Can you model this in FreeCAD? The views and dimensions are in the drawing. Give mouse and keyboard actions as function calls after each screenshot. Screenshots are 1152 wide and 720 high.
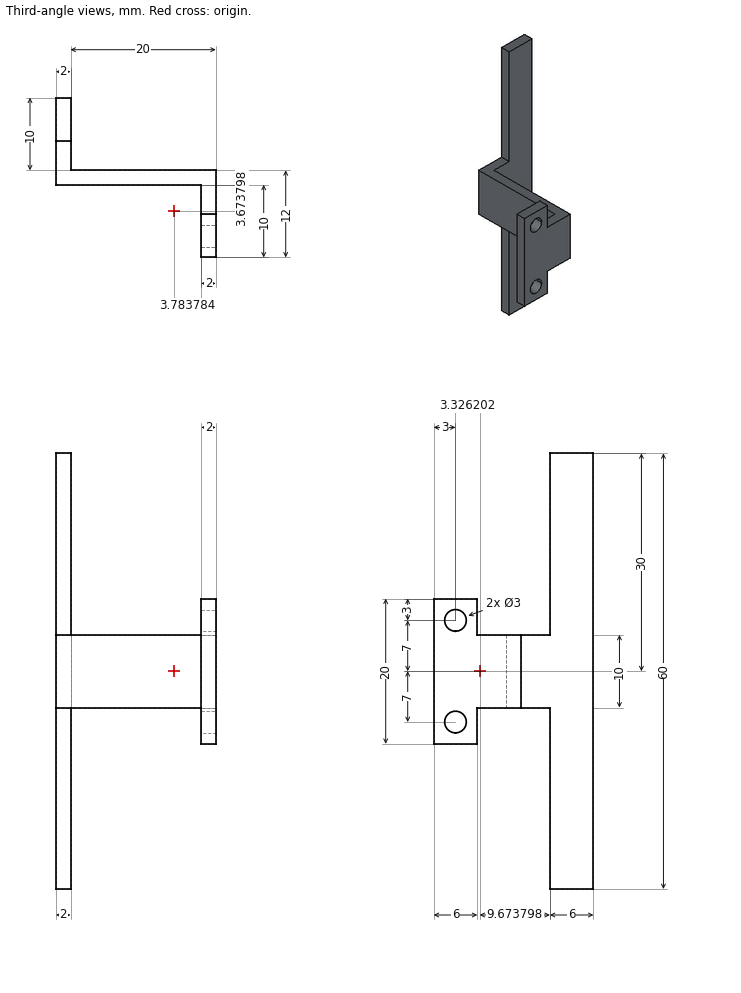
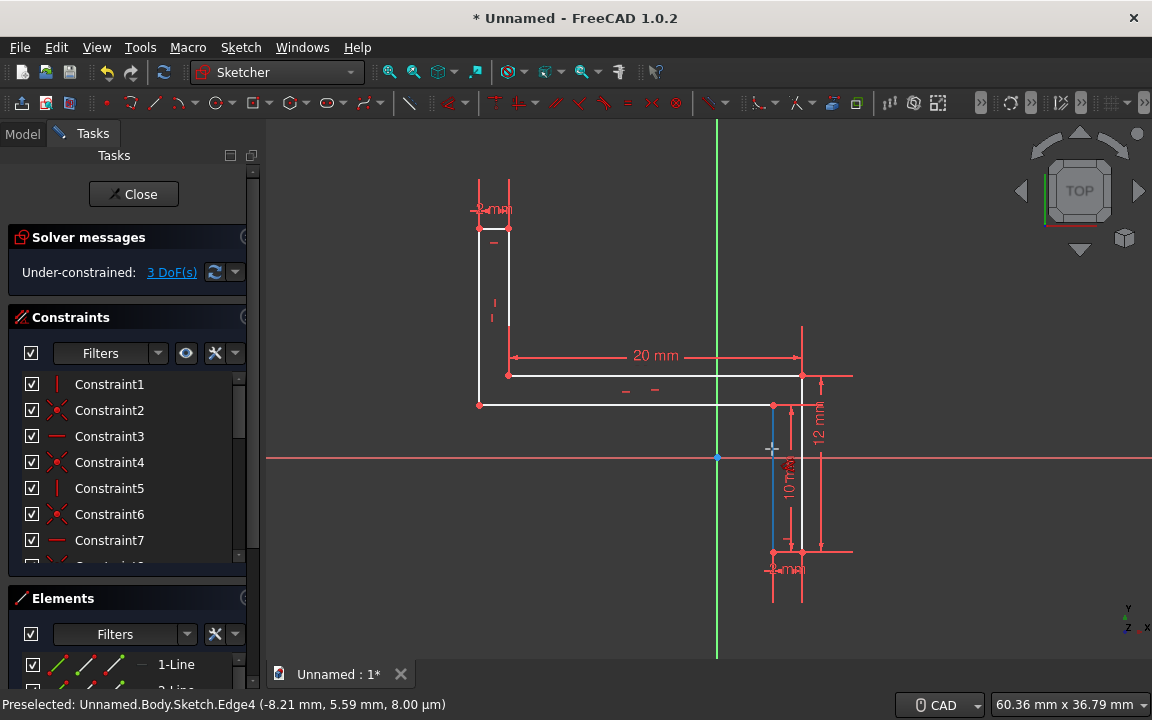
click(509, 332)
click(543, 302)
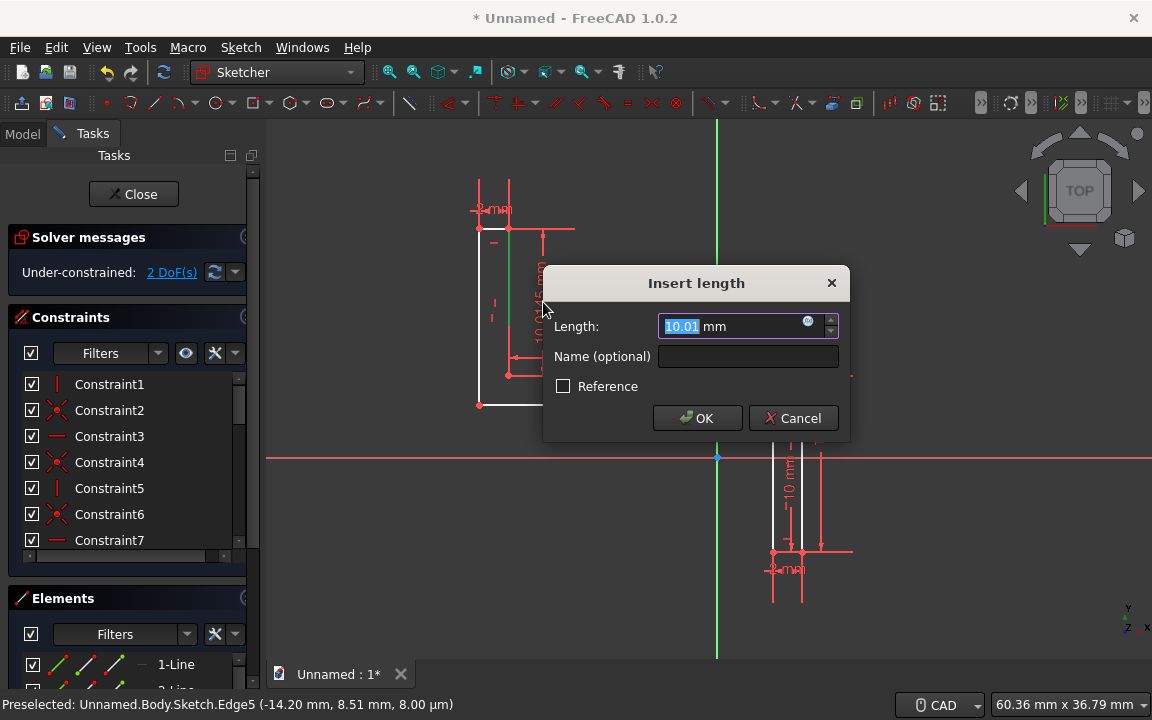
text(10)
key(Return)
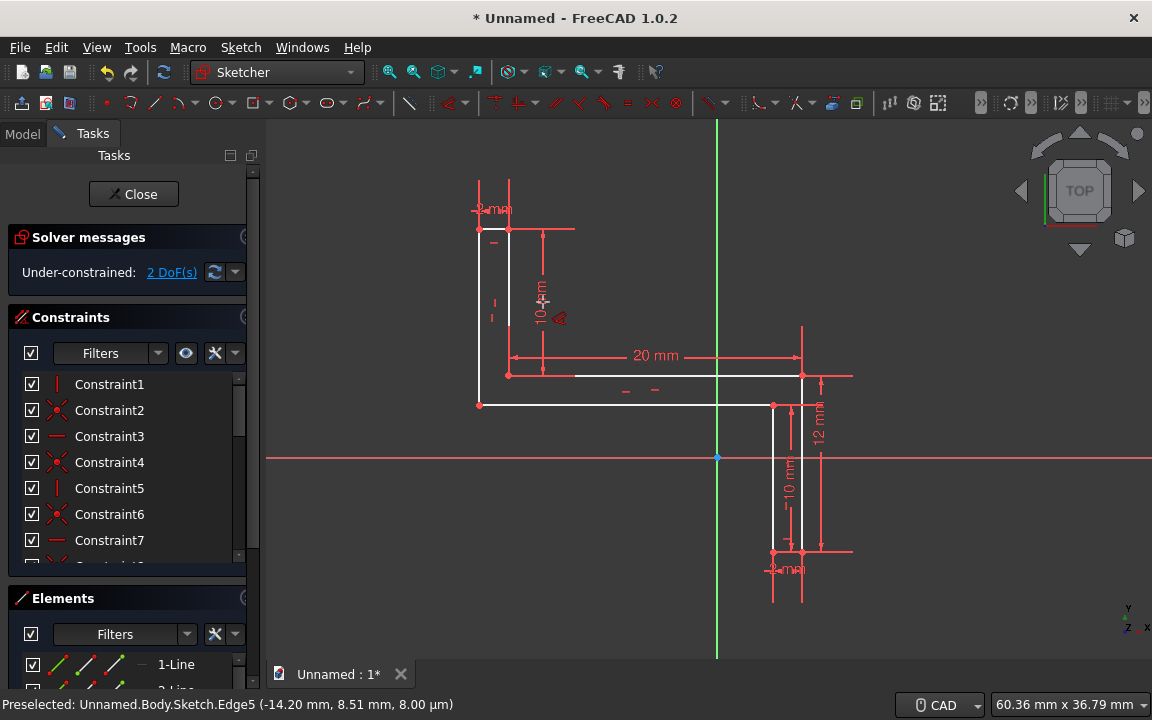
click(773, 405)
click(745, 516)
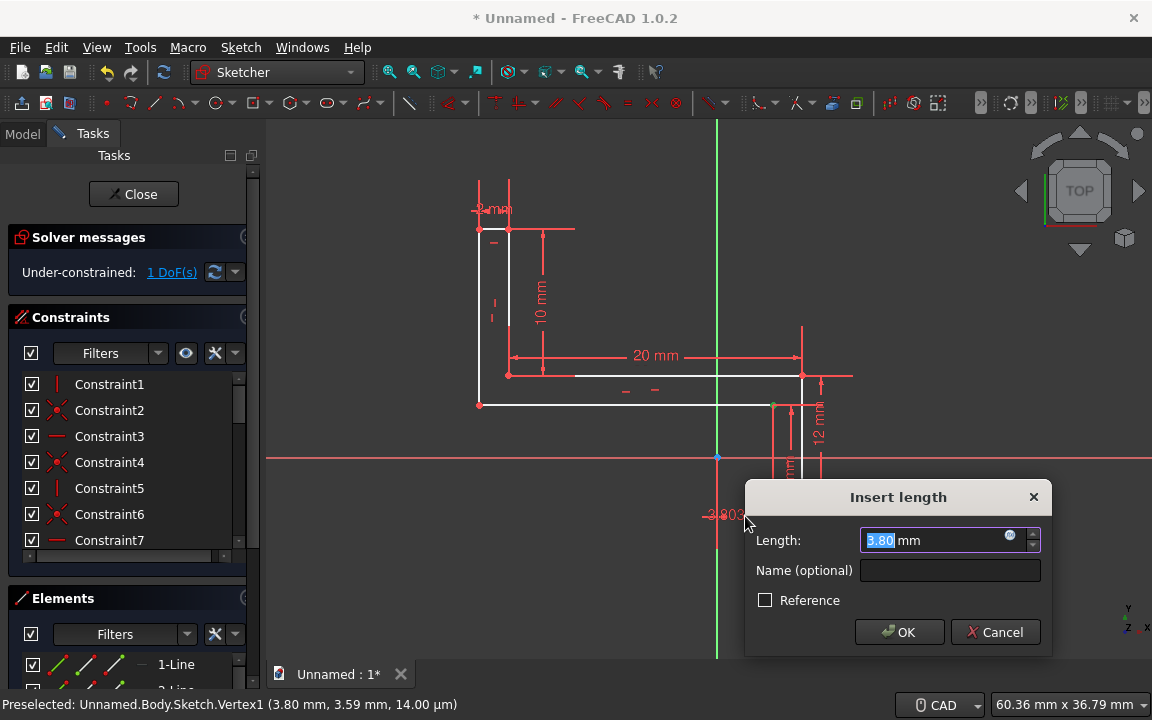
text(3.783784)
key(Return)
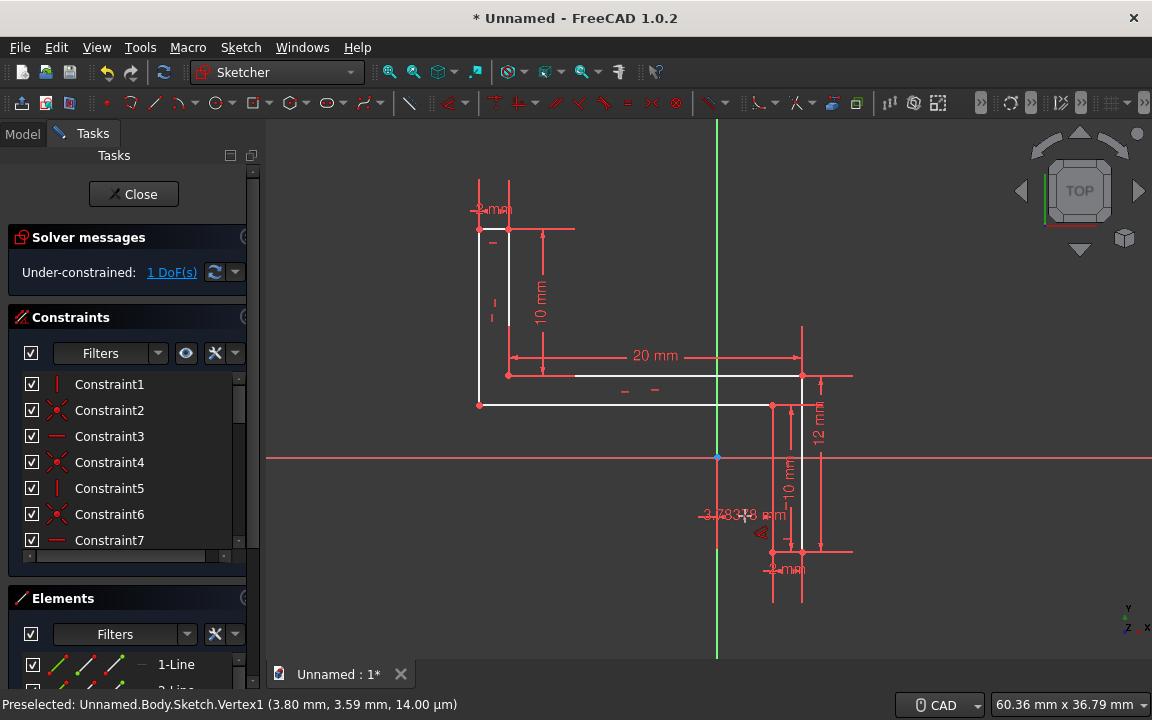
click(773, 405)
click(683, 432)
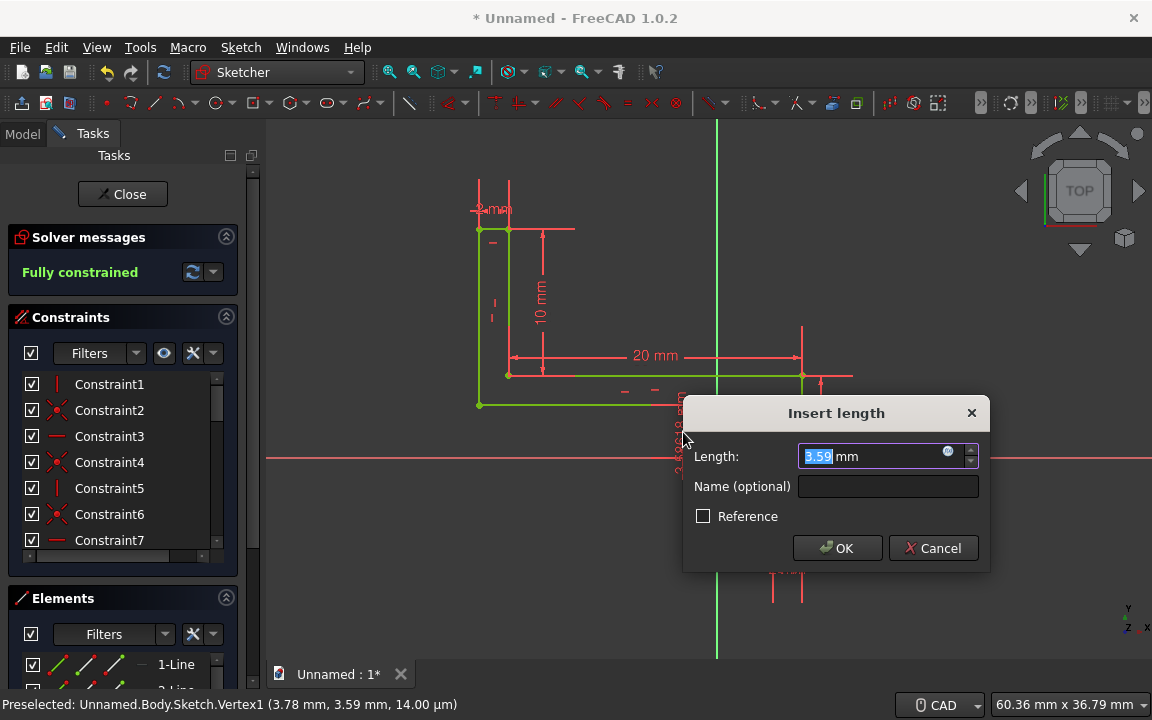
text(3.673798)
key(Return)
key(Escape)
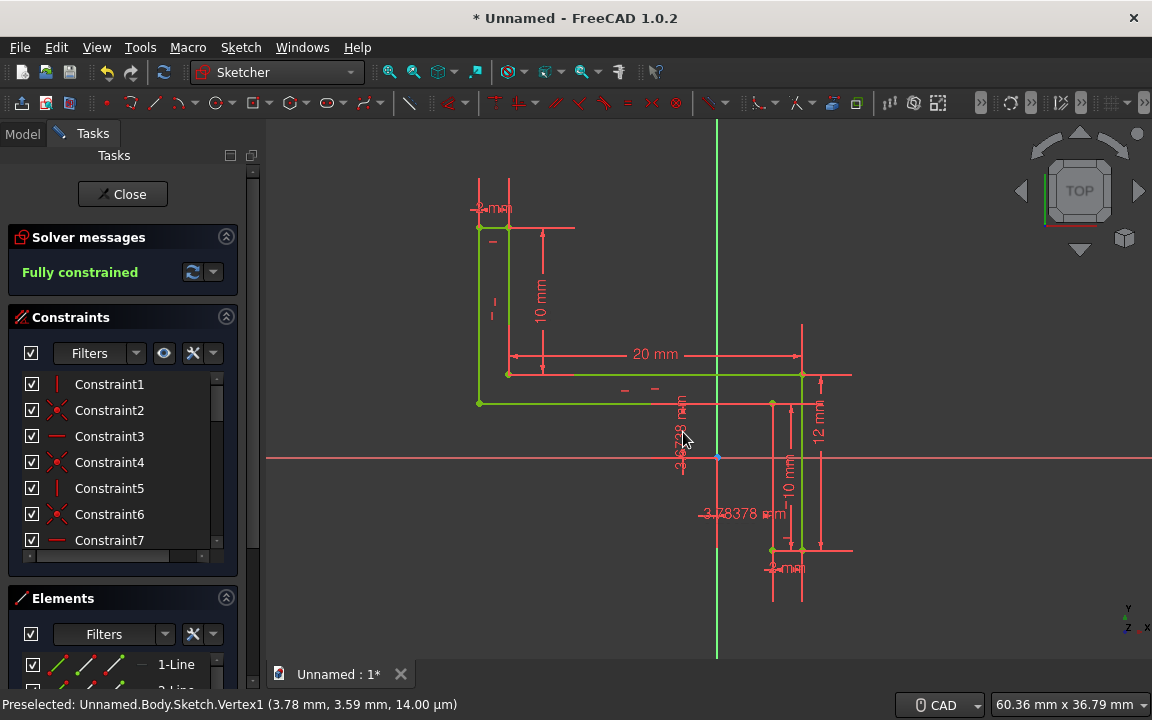
click(123, 194)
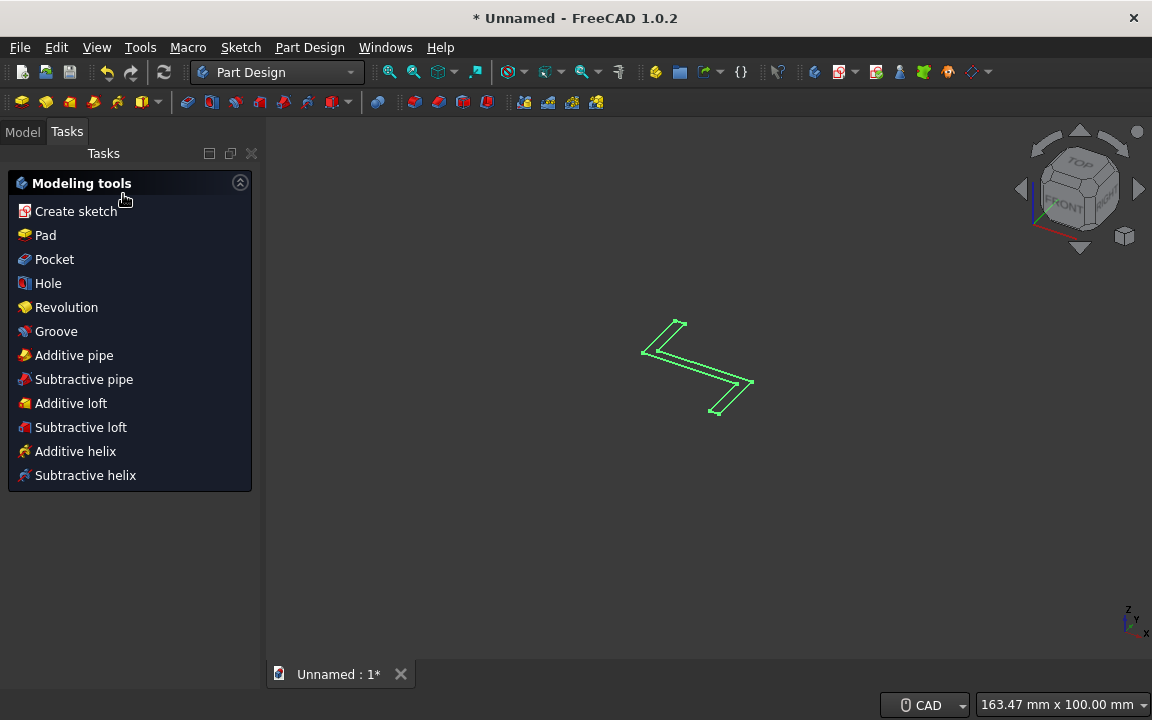
click(22, 102)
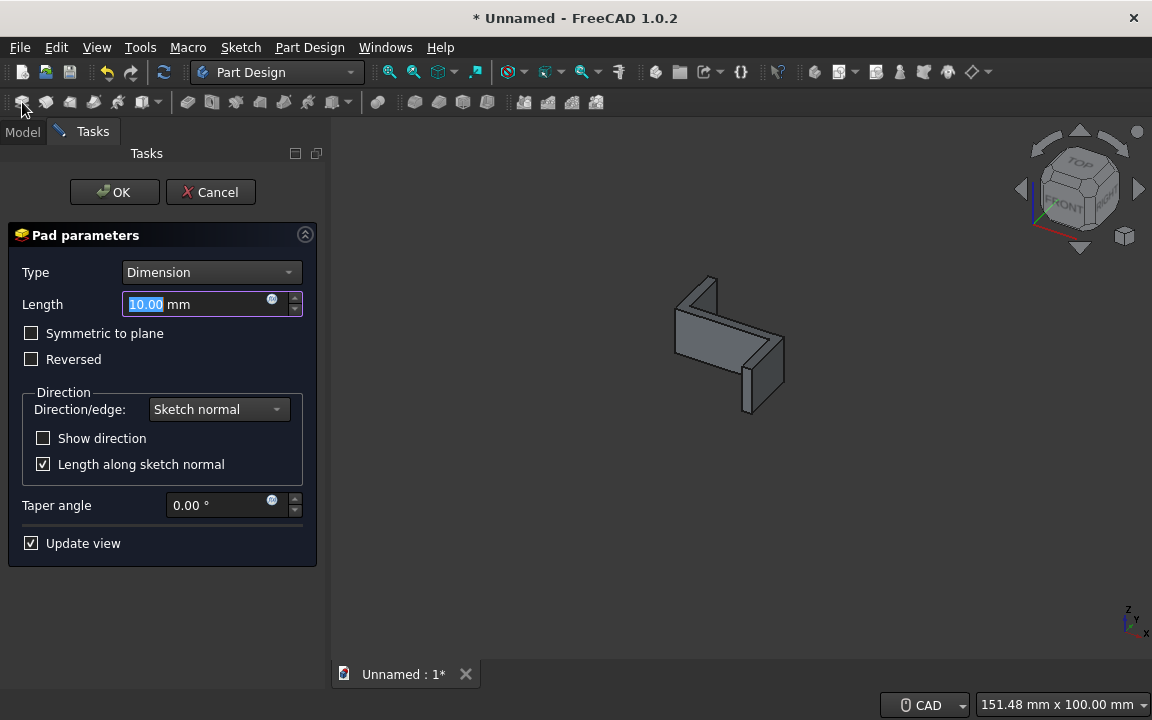
text(10)
key(Tab)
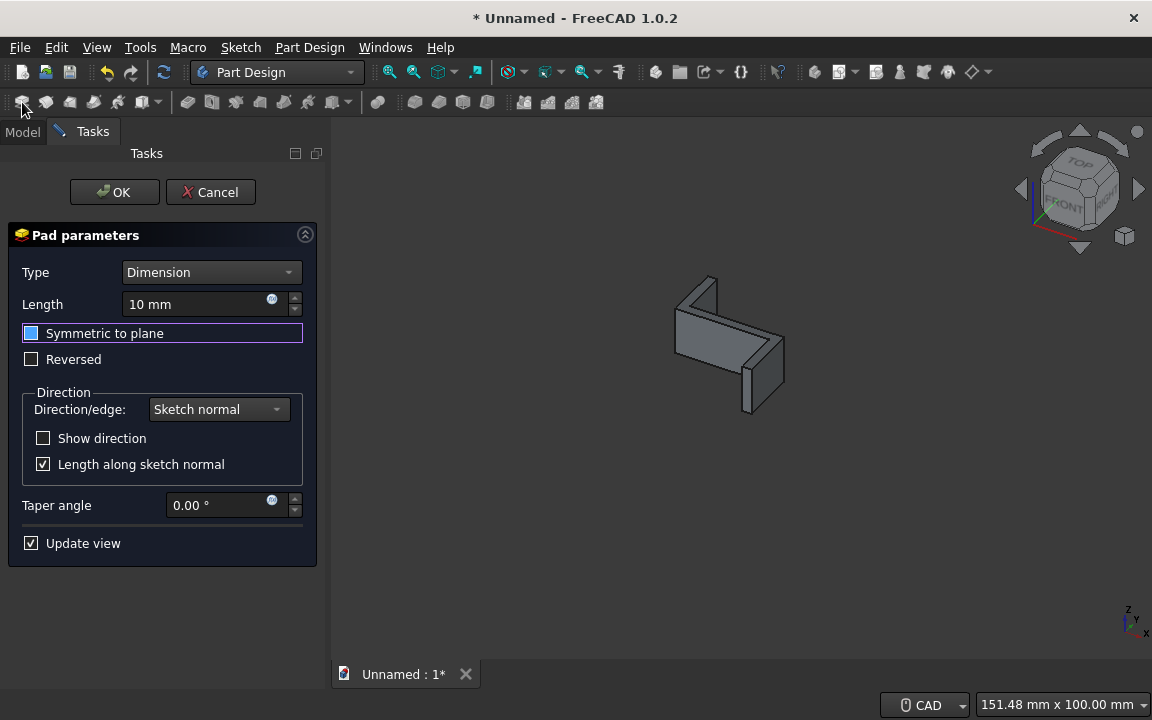
click(30, 333)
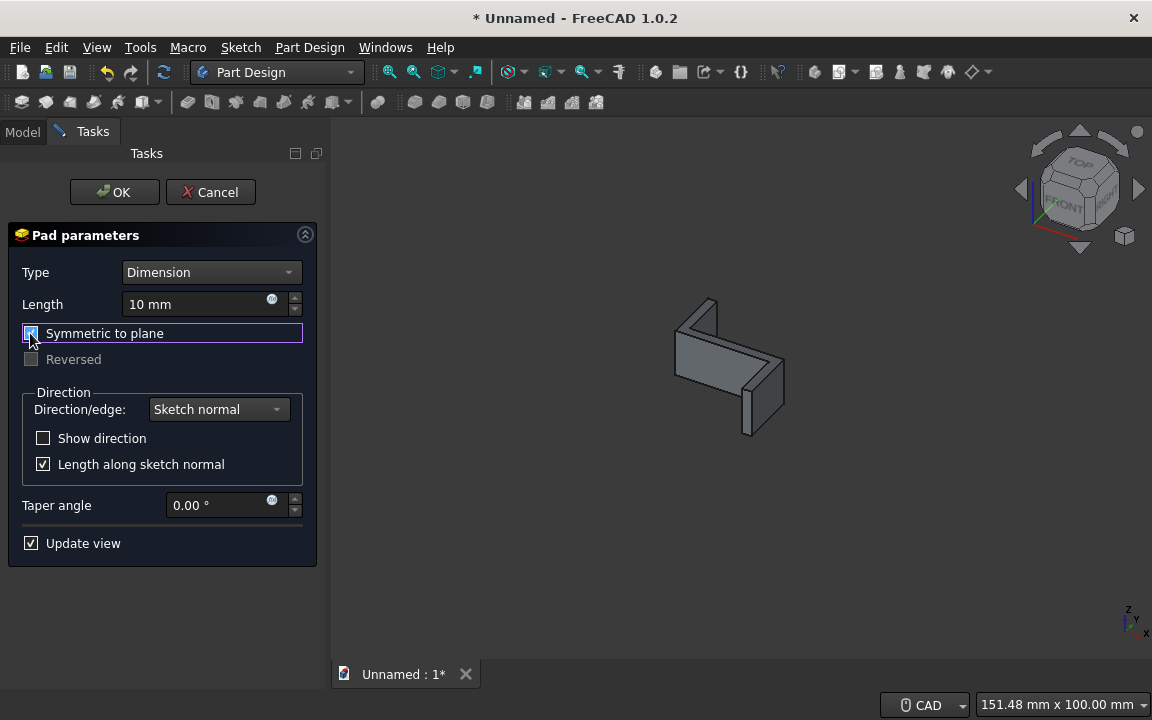
click(115, 192)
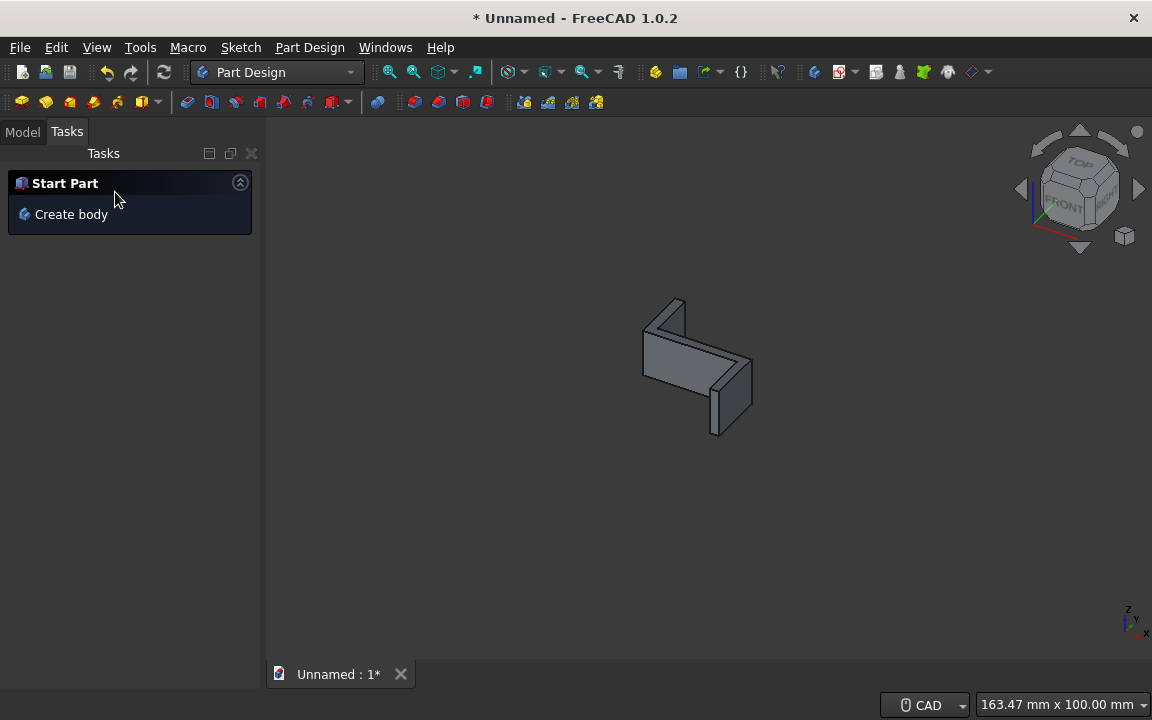
click(390, 72)